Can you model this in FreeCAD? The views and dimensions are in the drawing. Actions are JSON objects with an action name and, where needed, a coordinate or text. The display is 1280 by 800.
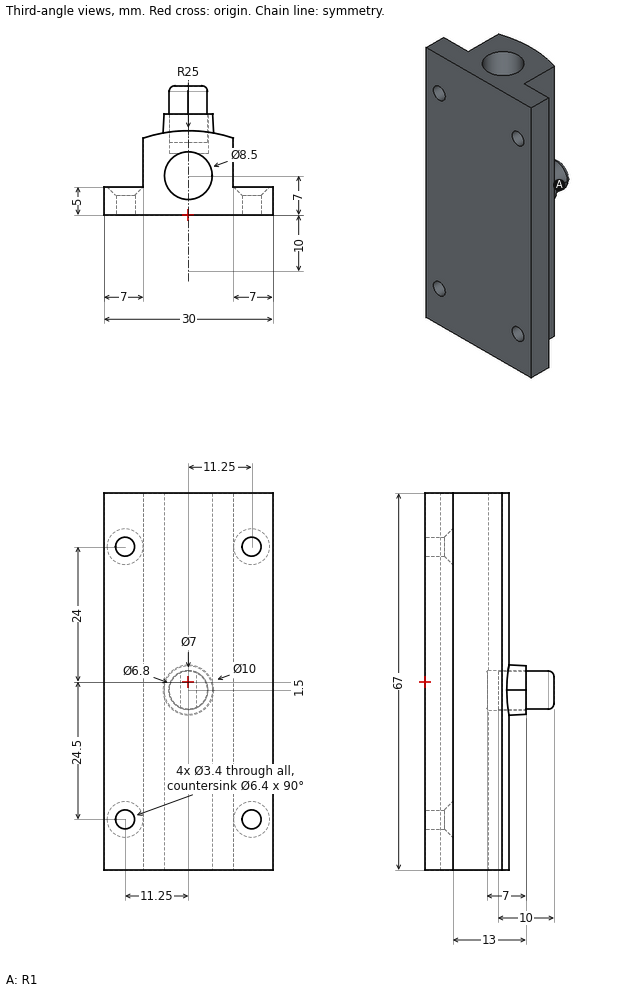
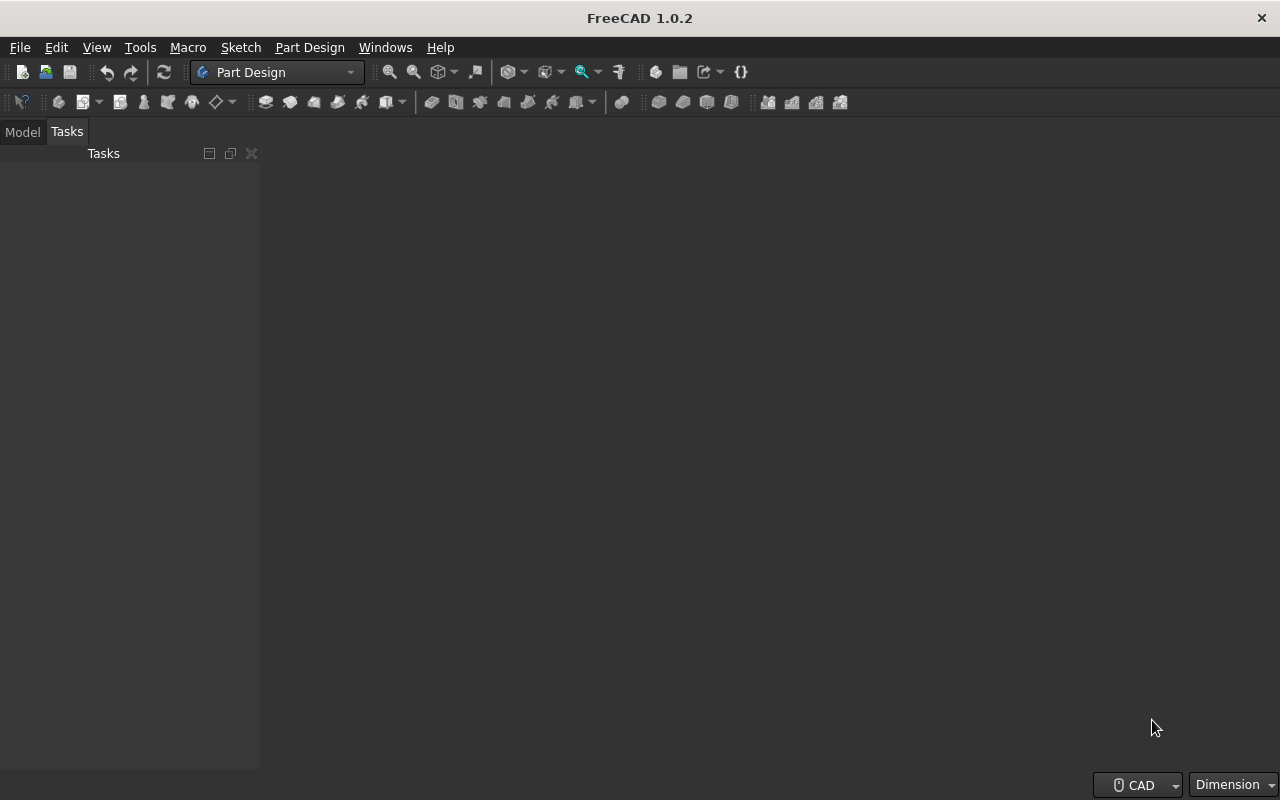
{"action": "key", "text": "ctrl+n"}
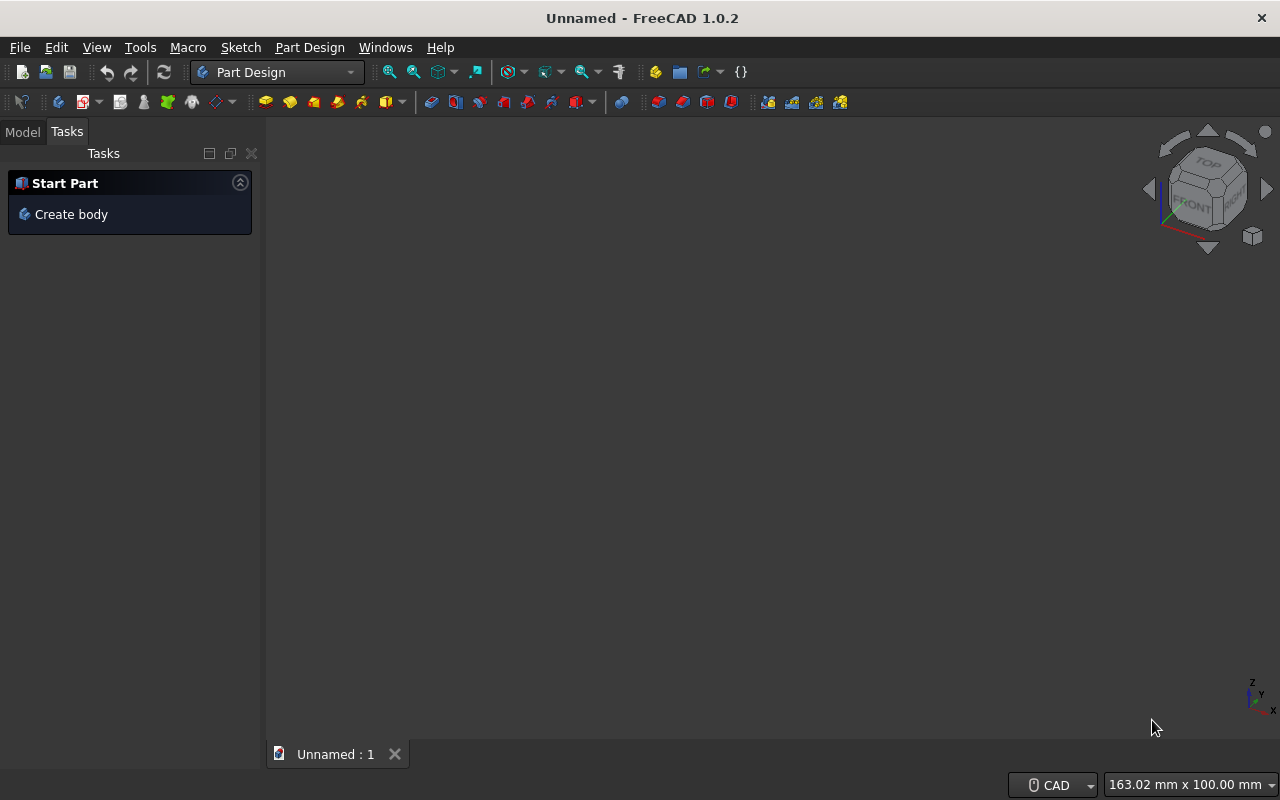
{"action": "left_click", "coordinate": [84, 102]}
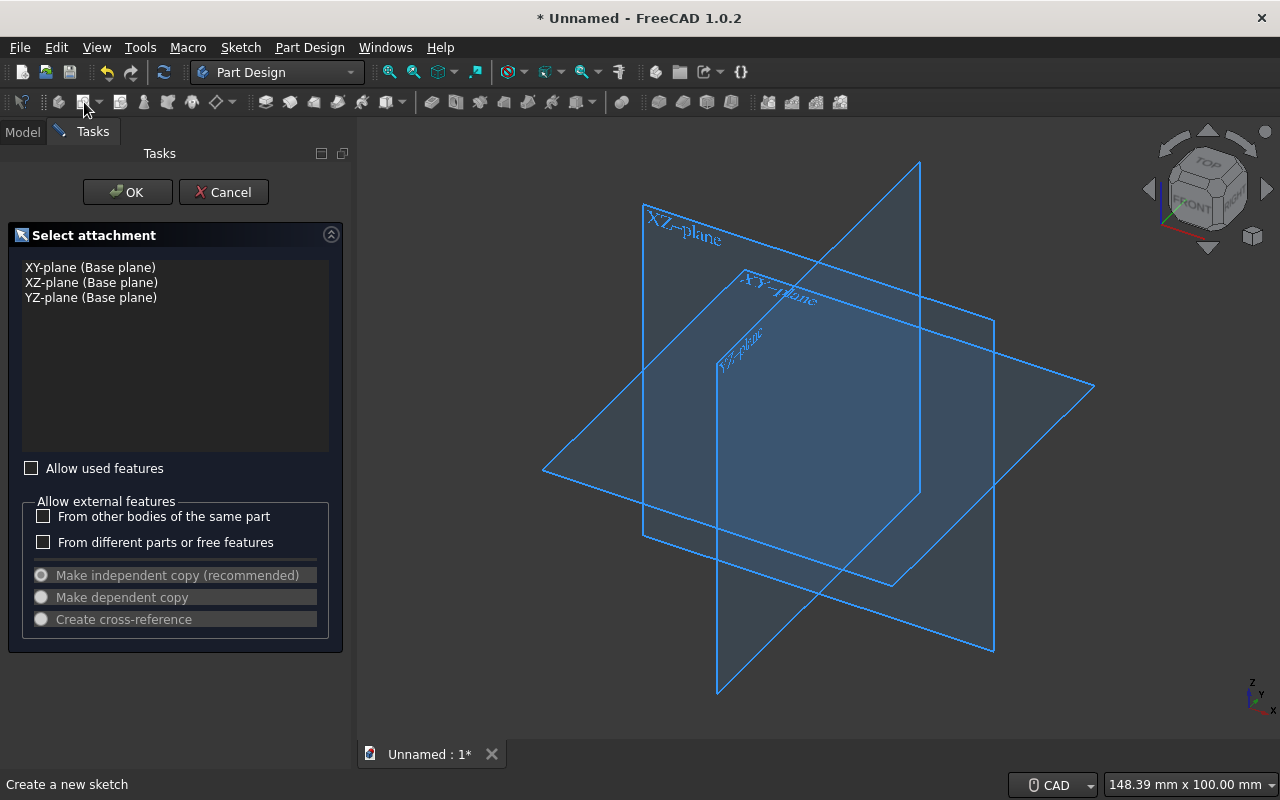
{"action": "left_click", "coordinate": [82, 268]}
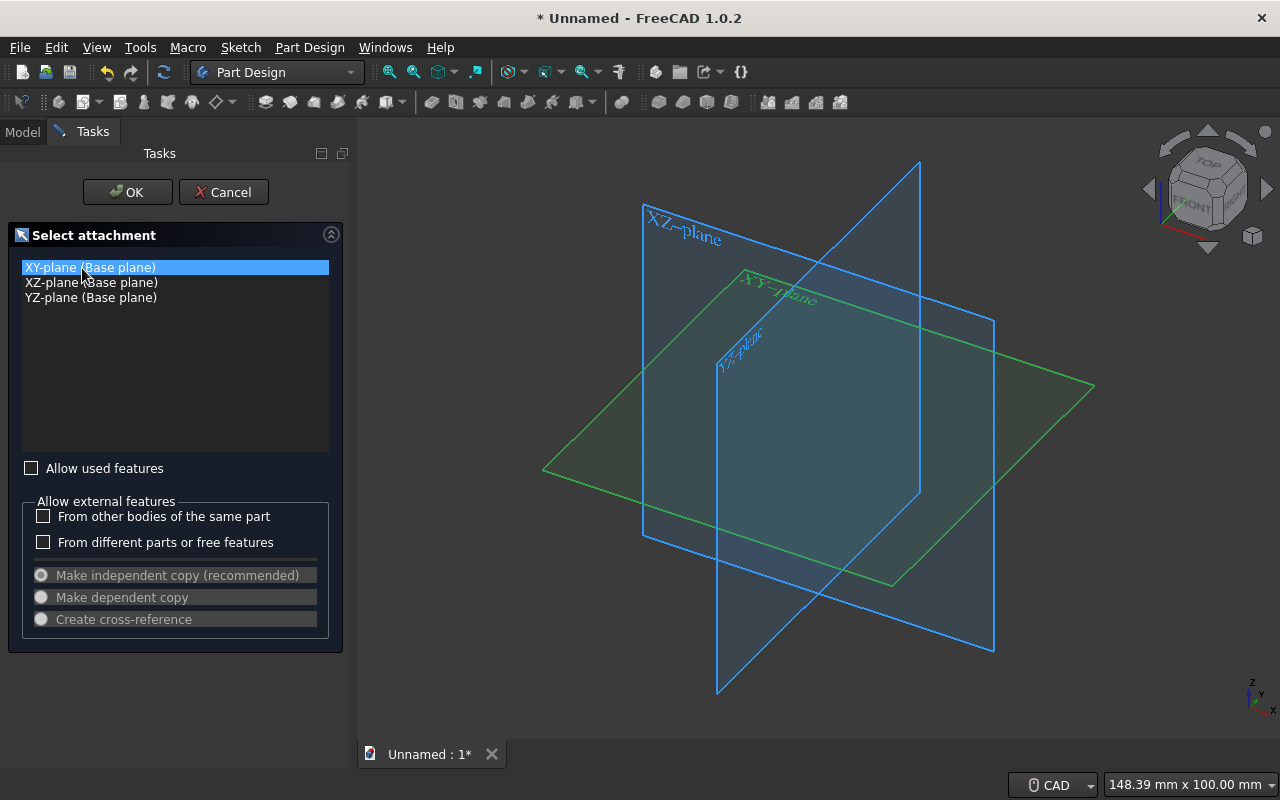
{"action": "left_click", "coordinate": [128, 192]}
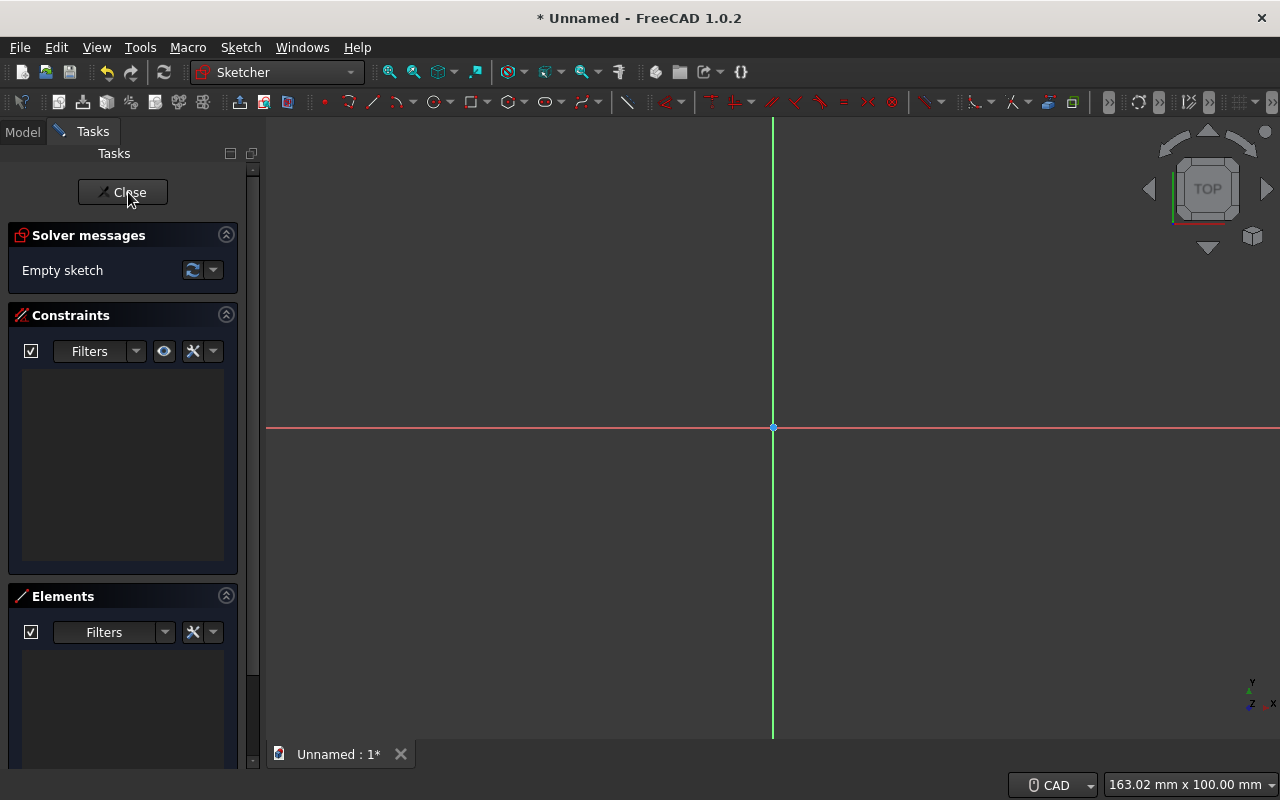
{"action": "scroll", "coordinate": [803, 361], "scroll_direction": "up", "scroll_amount": 6}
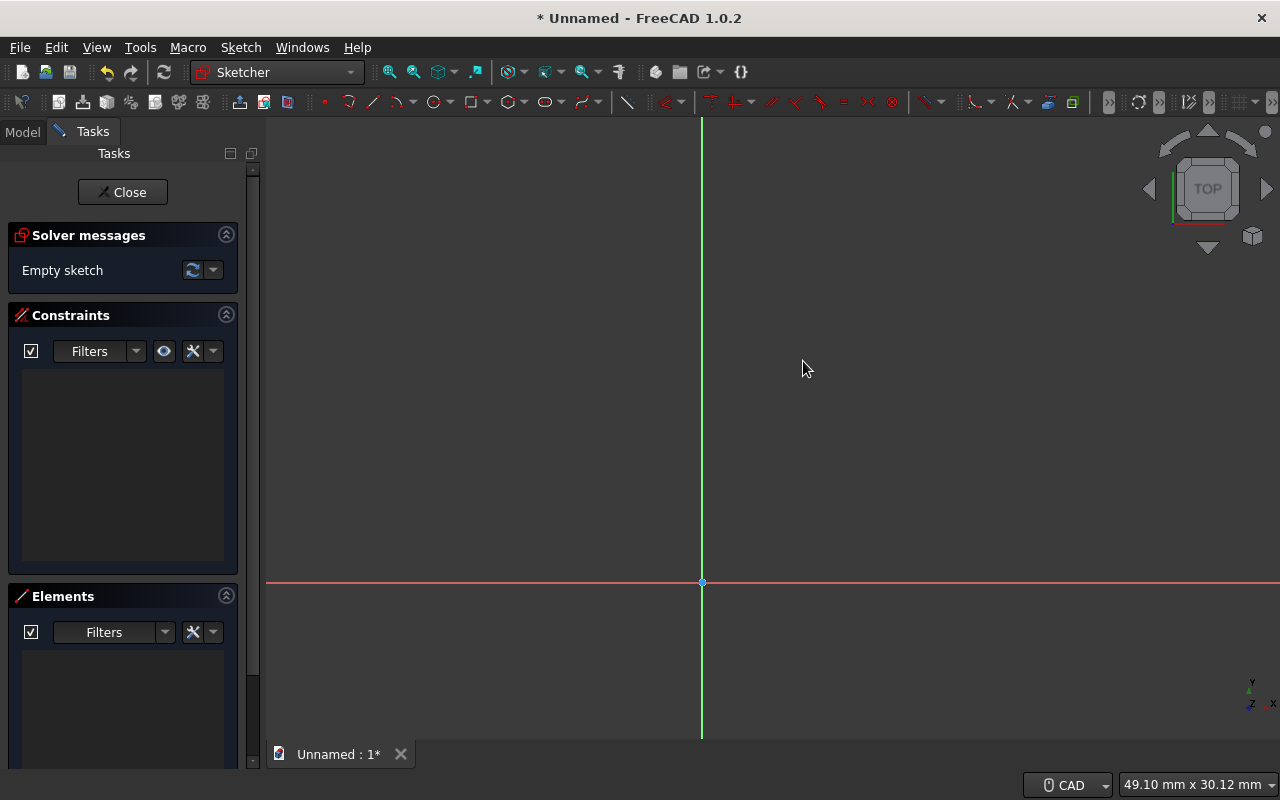
{"action": "key", "text": "g m"}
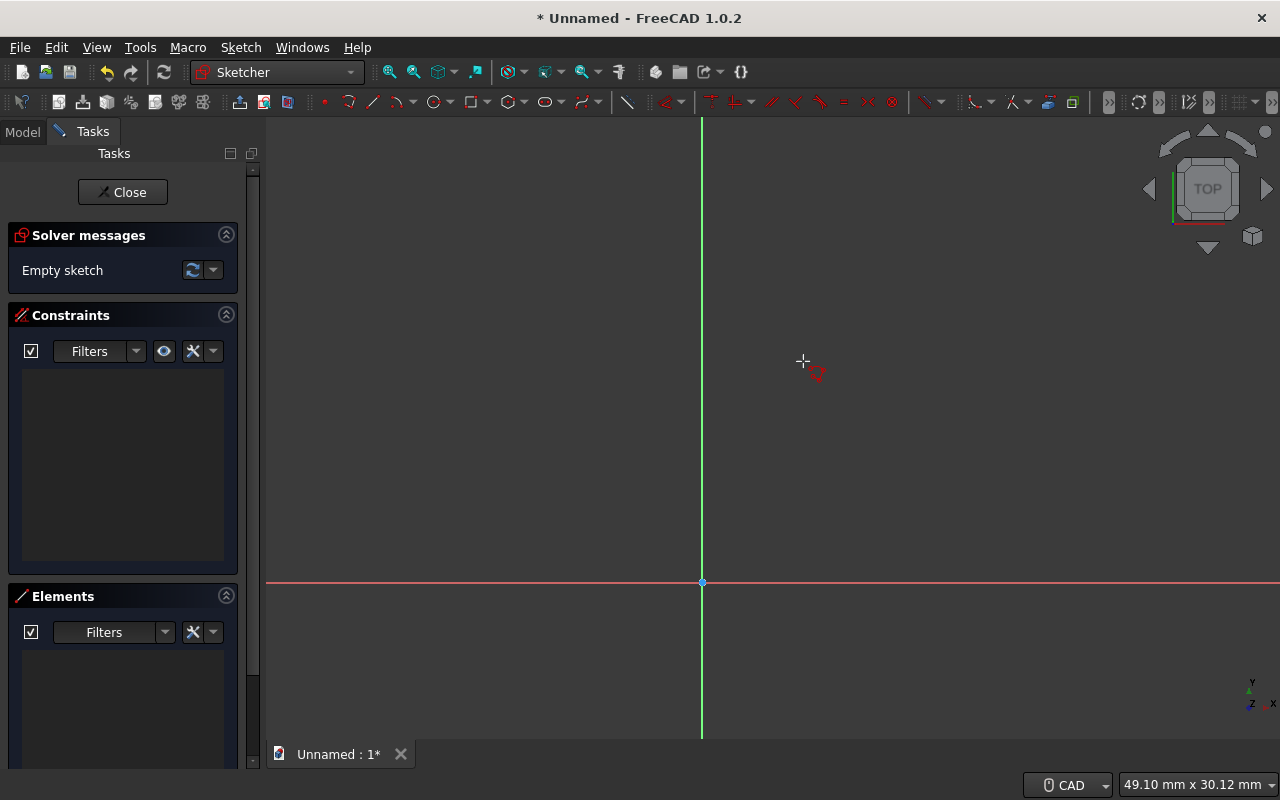
{"action": "left_click", "coordinate": [537, 300]}
{"action": "left_click", "coordinate": [537, 479]}
{"action": "left_click", "coordinate": [392, 479]}
{"action": "left_click", "coordinate": [392, 583]}
{"action": "left_click", "coordinate": [1012, 574]}
{"action": "left_click", "coordinate": [1012, 479]}
{"action": "left_click", "coordinate": [867, 479]}
{"action": "left_click", "coordinate": [867, 300]}
{"action": "right_click", "coordinate": [867, 300]}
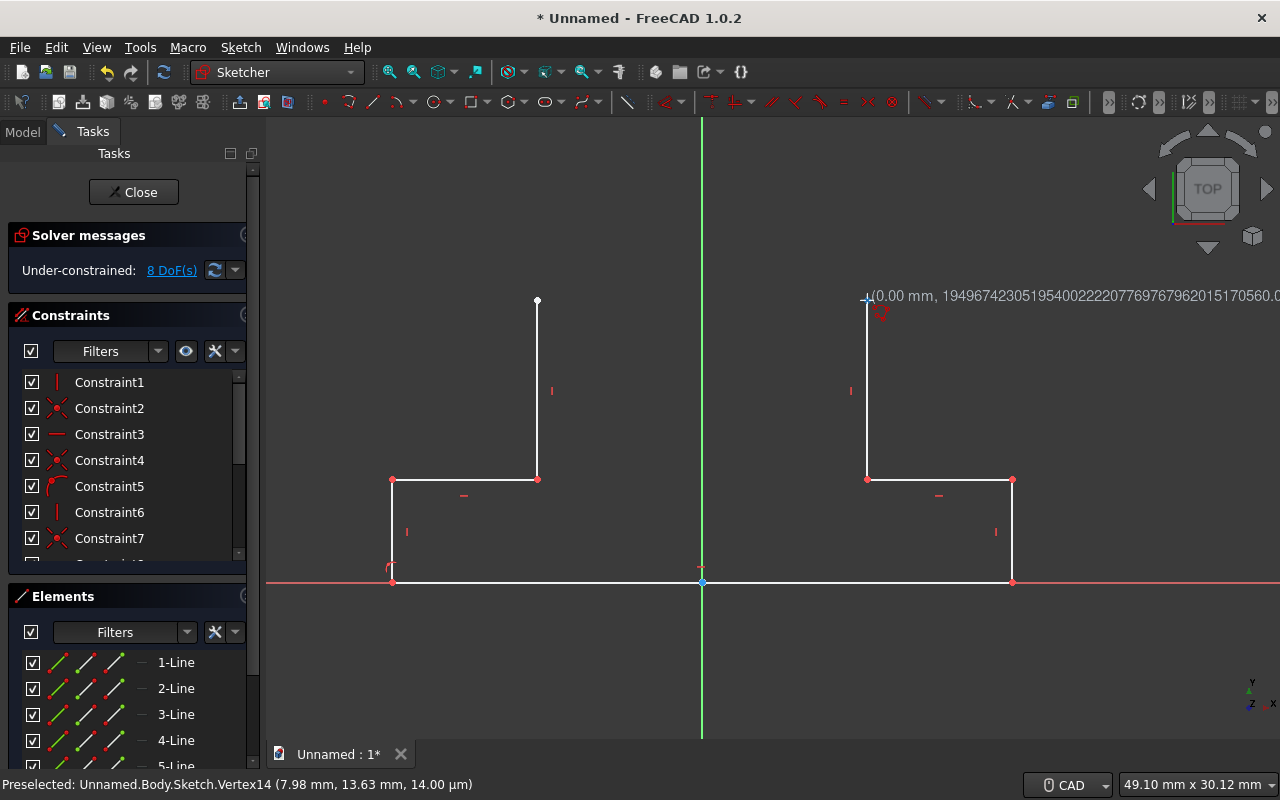
{"action": "key", "text": "g 3 a"}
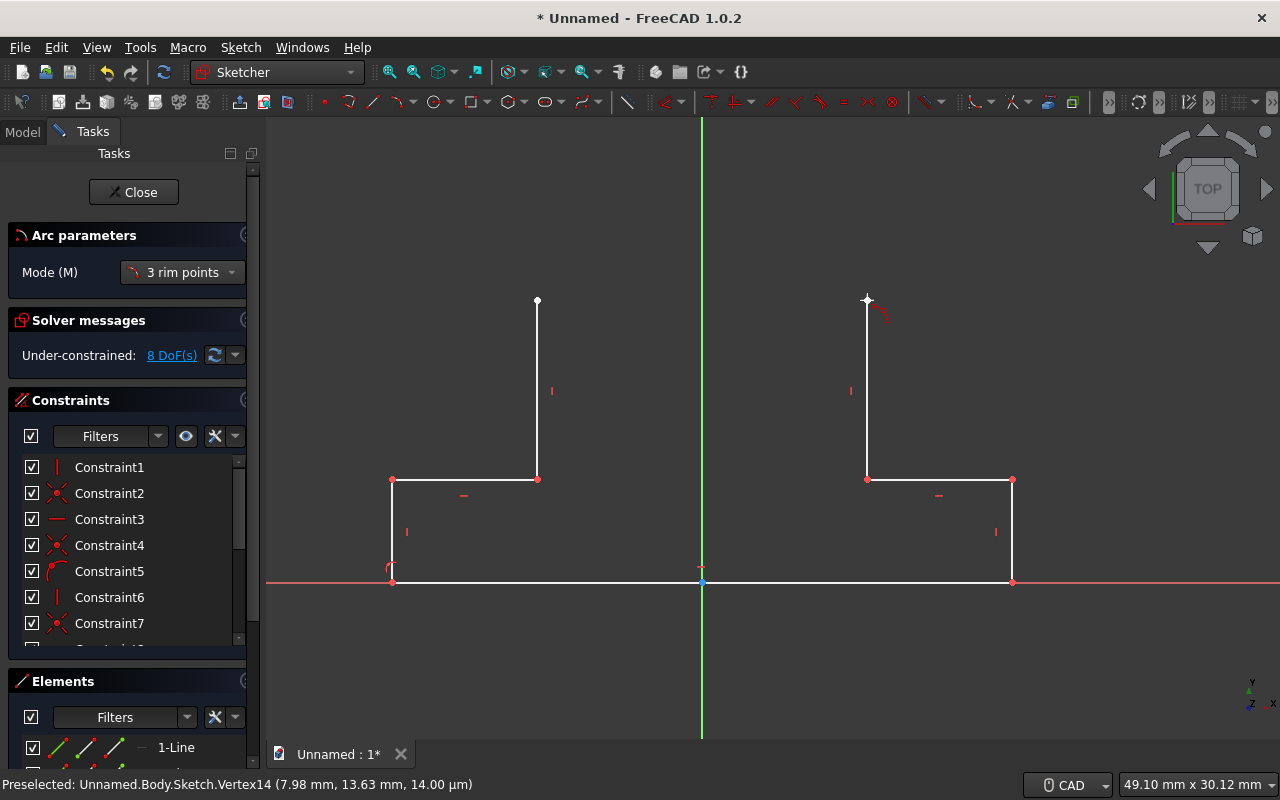
{"action": "left_click", "coordinate": [867, 301]}
{"action": "left_click", "coordinate": [537, 301]}
{"action": "left_click", "coordinate": [736, 274]}
{"action": "key", "text": "Escape"}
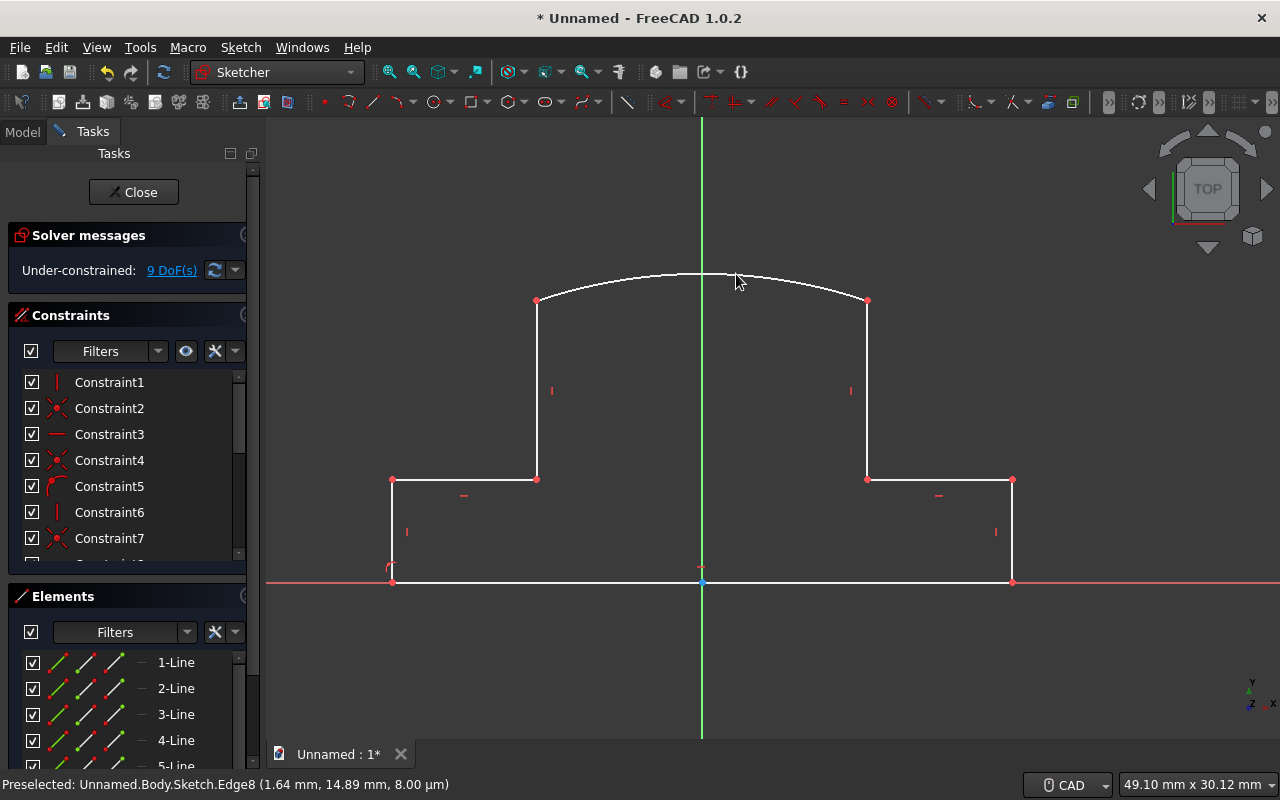
{"action": "scroll", "coordinate": [715, 145], "scroll_direction": "down", "scroll_amount": 1}